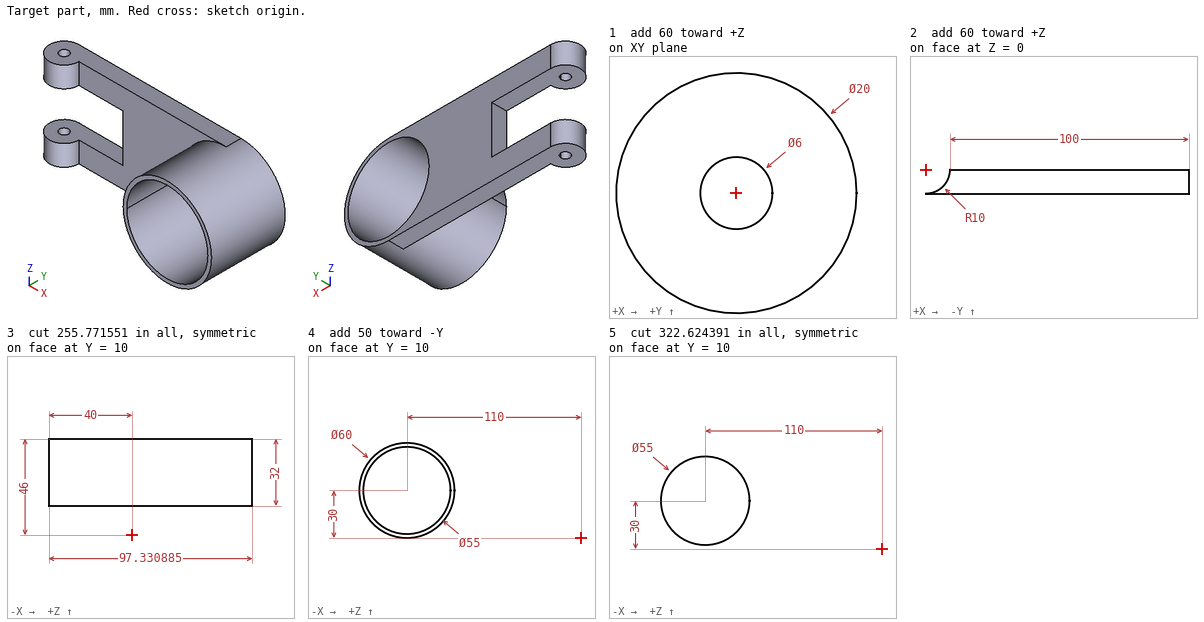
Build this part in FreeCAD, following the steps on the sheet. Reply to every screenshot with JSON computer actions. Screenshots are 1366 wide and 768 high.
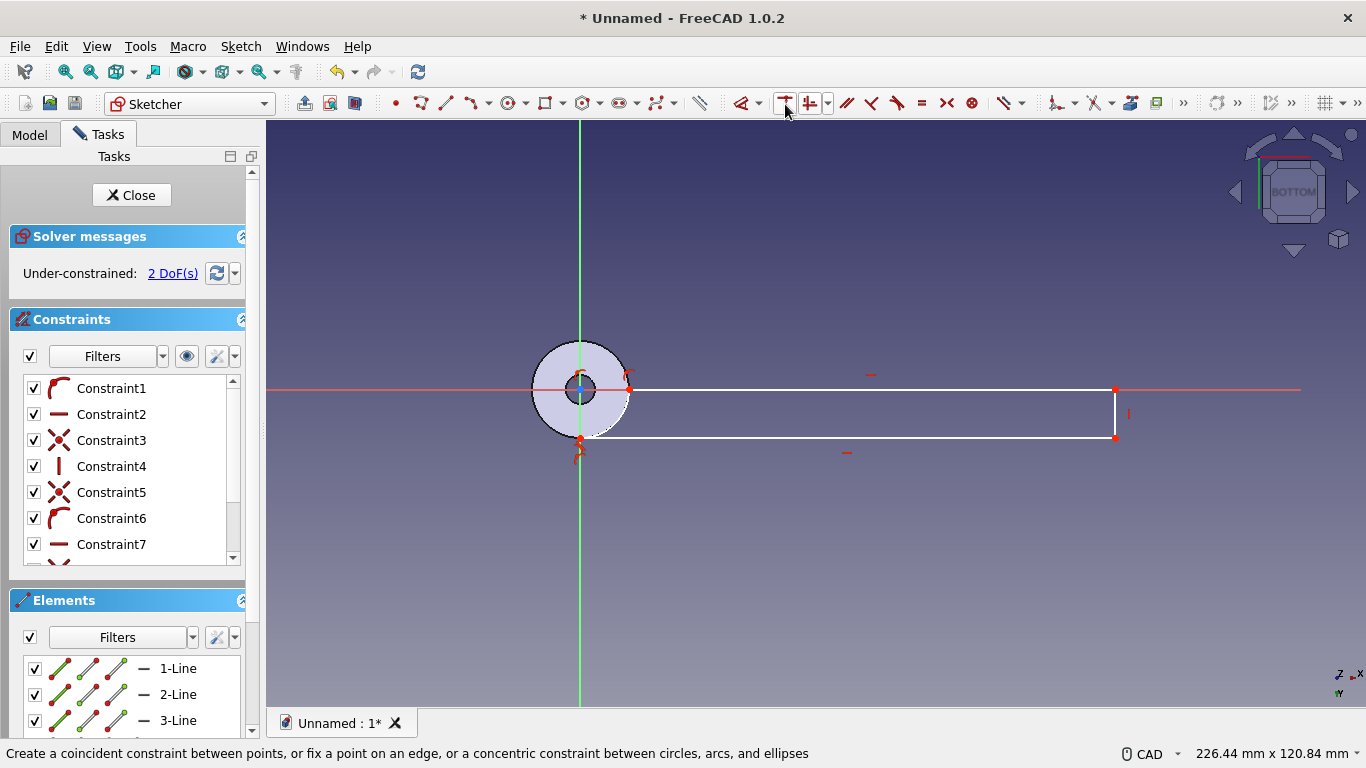
{"action": "left_click", "coordinate": [740, 104]}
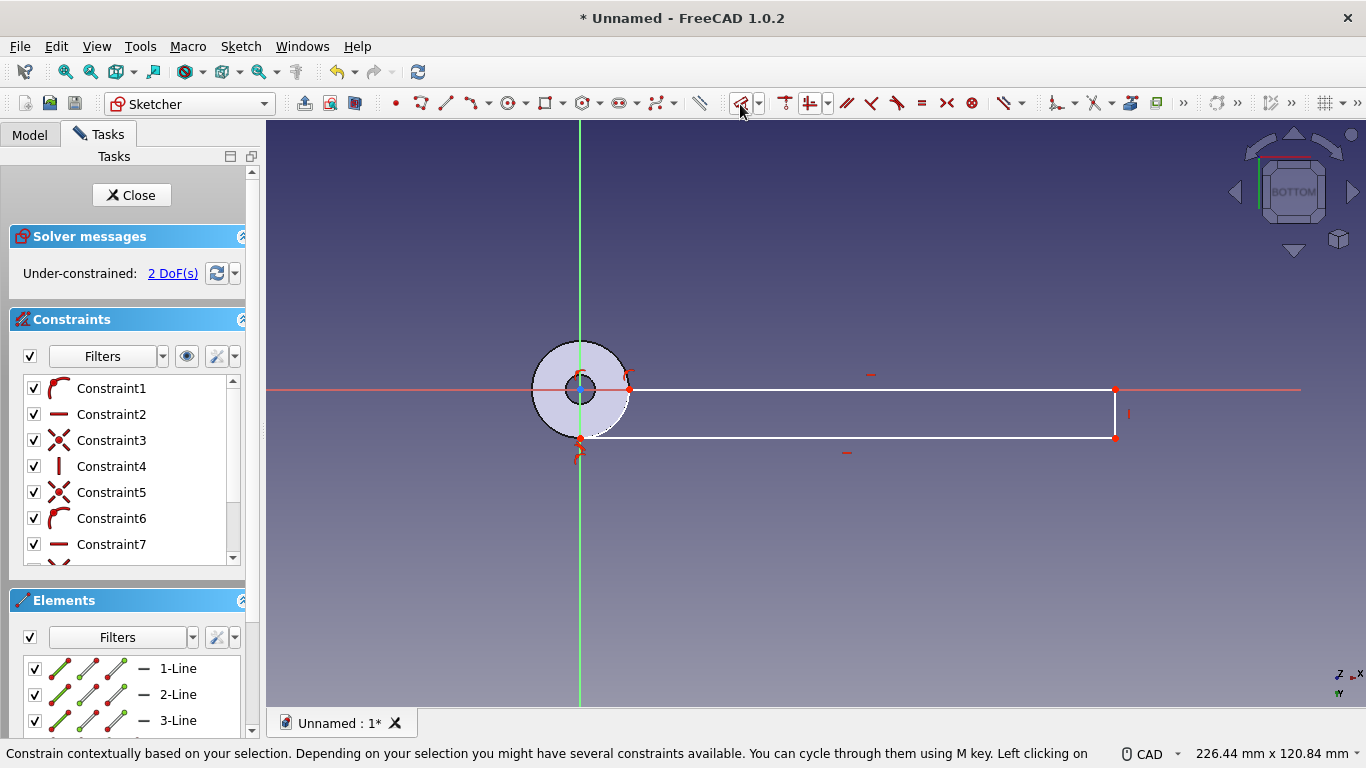
{"action": "left_click", "coordinate": [624, 412]}
{"action": "left_click", "coordinate": [626, 457]}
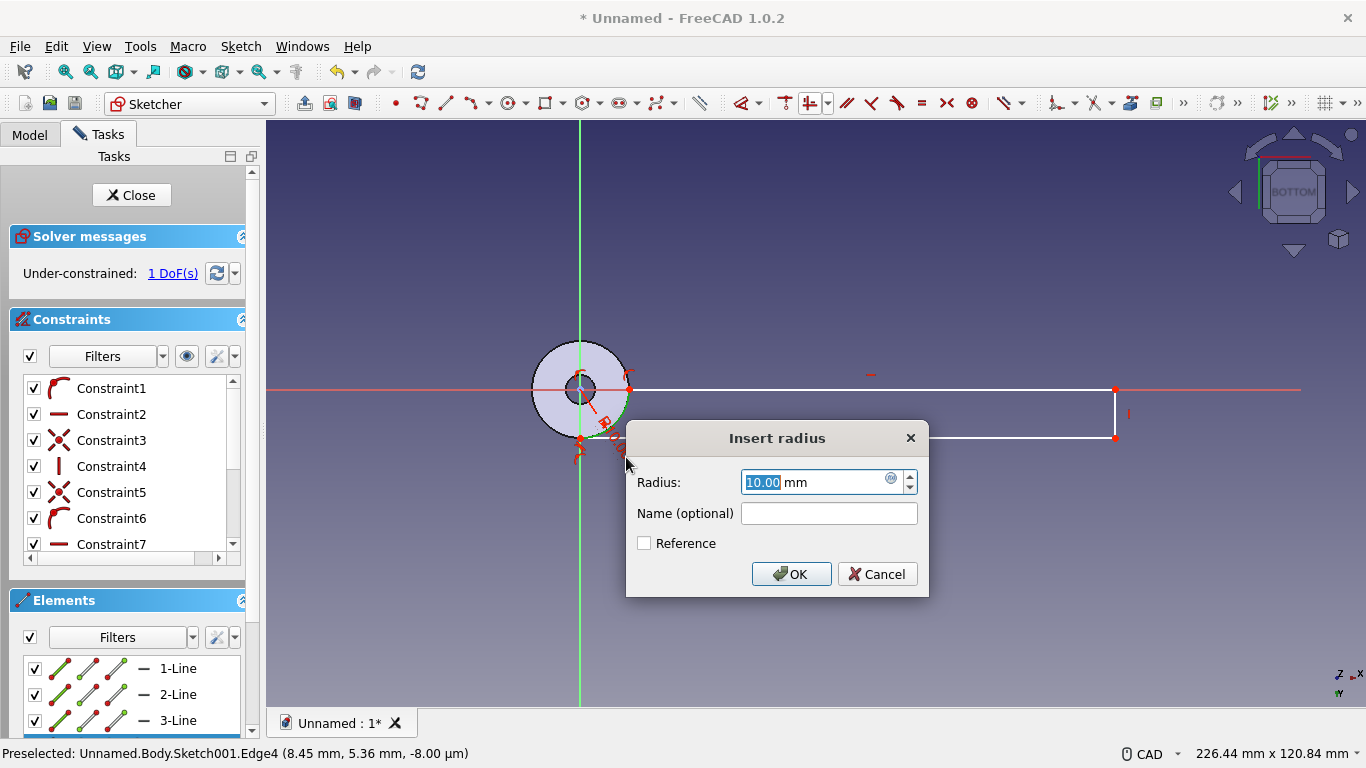
{"action": "type", "text": "10"}
{"action": "key", "text": "Return"}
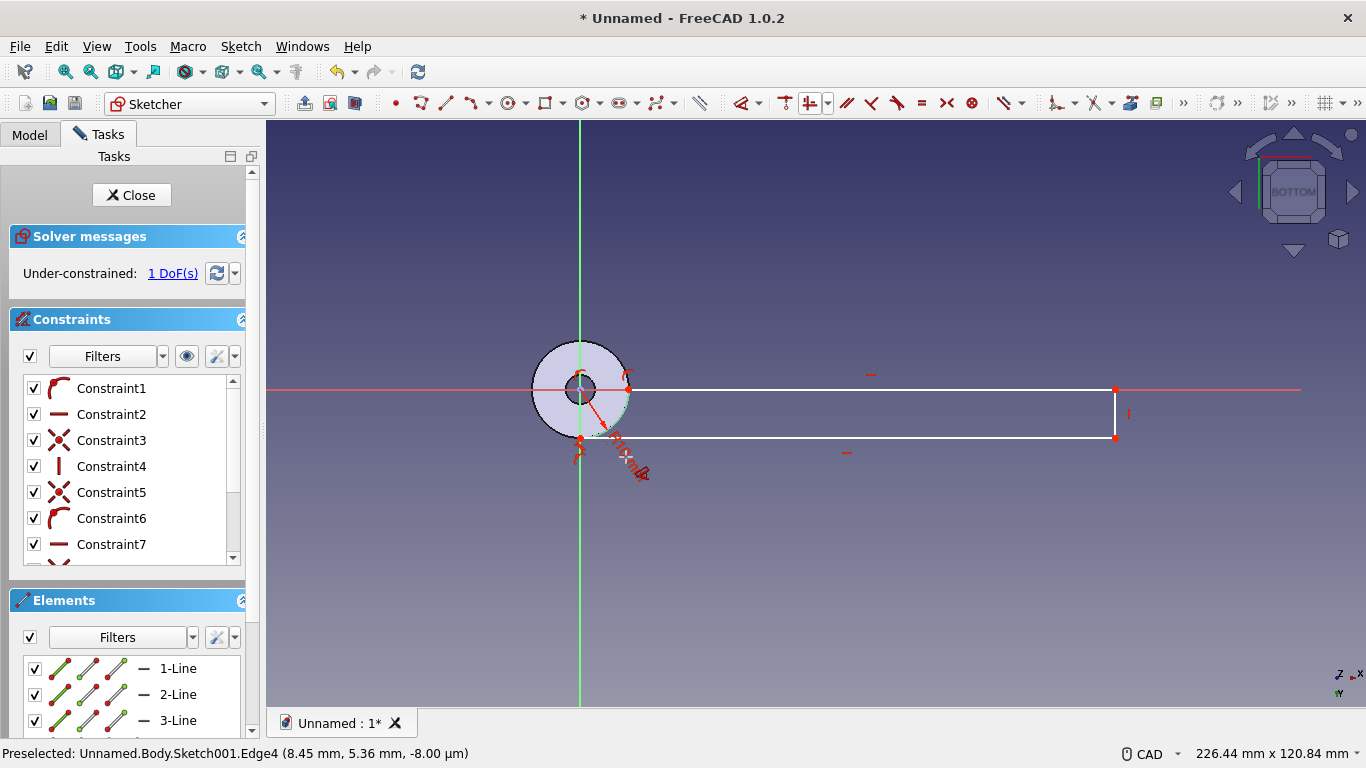
{"action": "left_click", "coordinate": [775, 390]}
{"action": "left_click", "coordinate": [872, 356]}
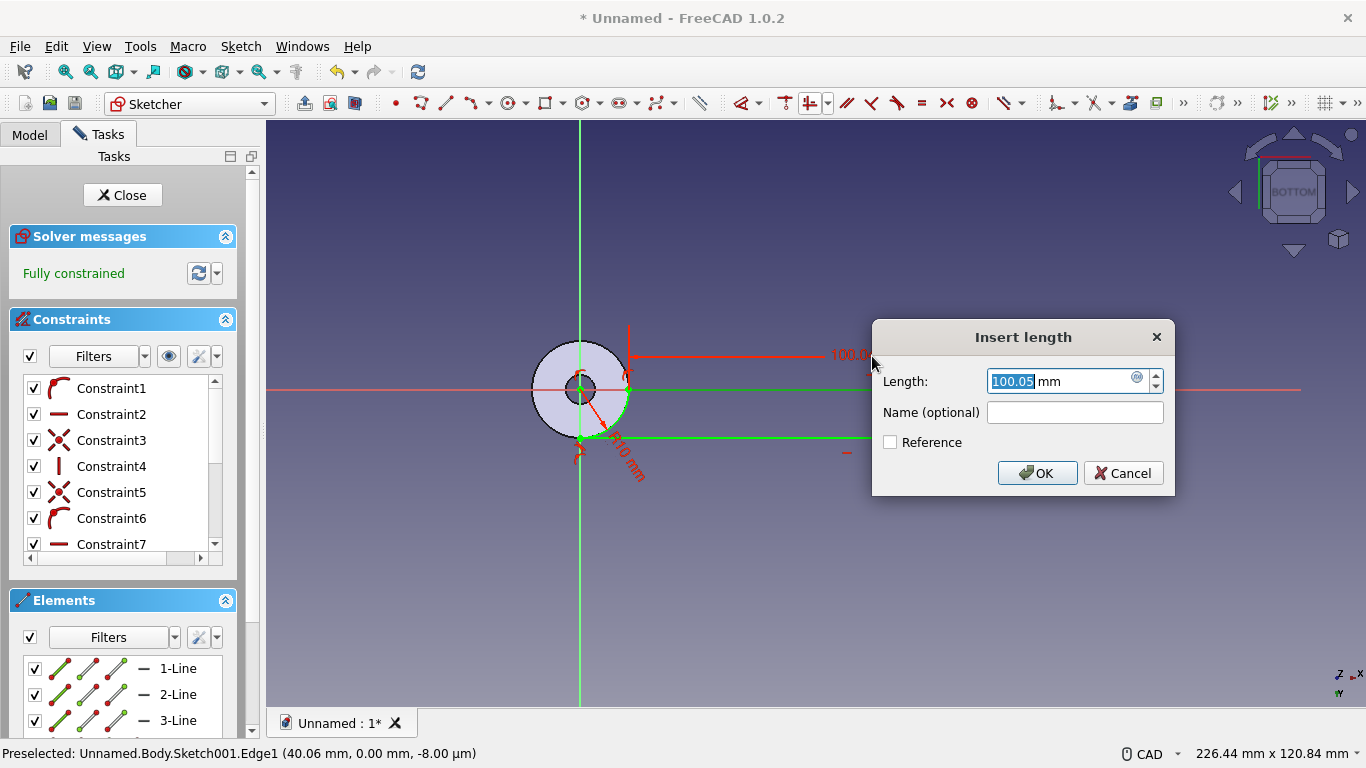
{"action": "type", "text": "100"}
{"action": "key", "text": "Return"}
{"action": "key", "text": "Escape"}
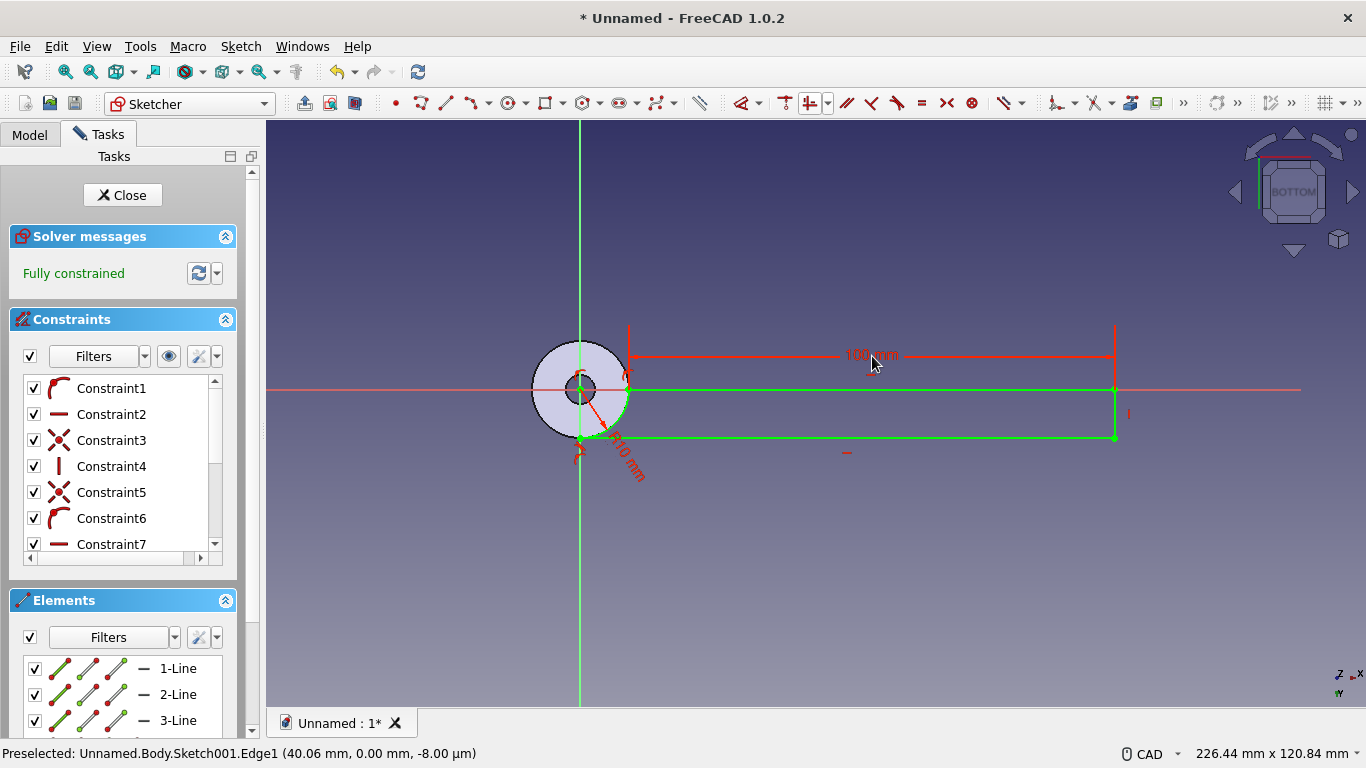
{"action": "left_click", "coordinate": [123, 195]}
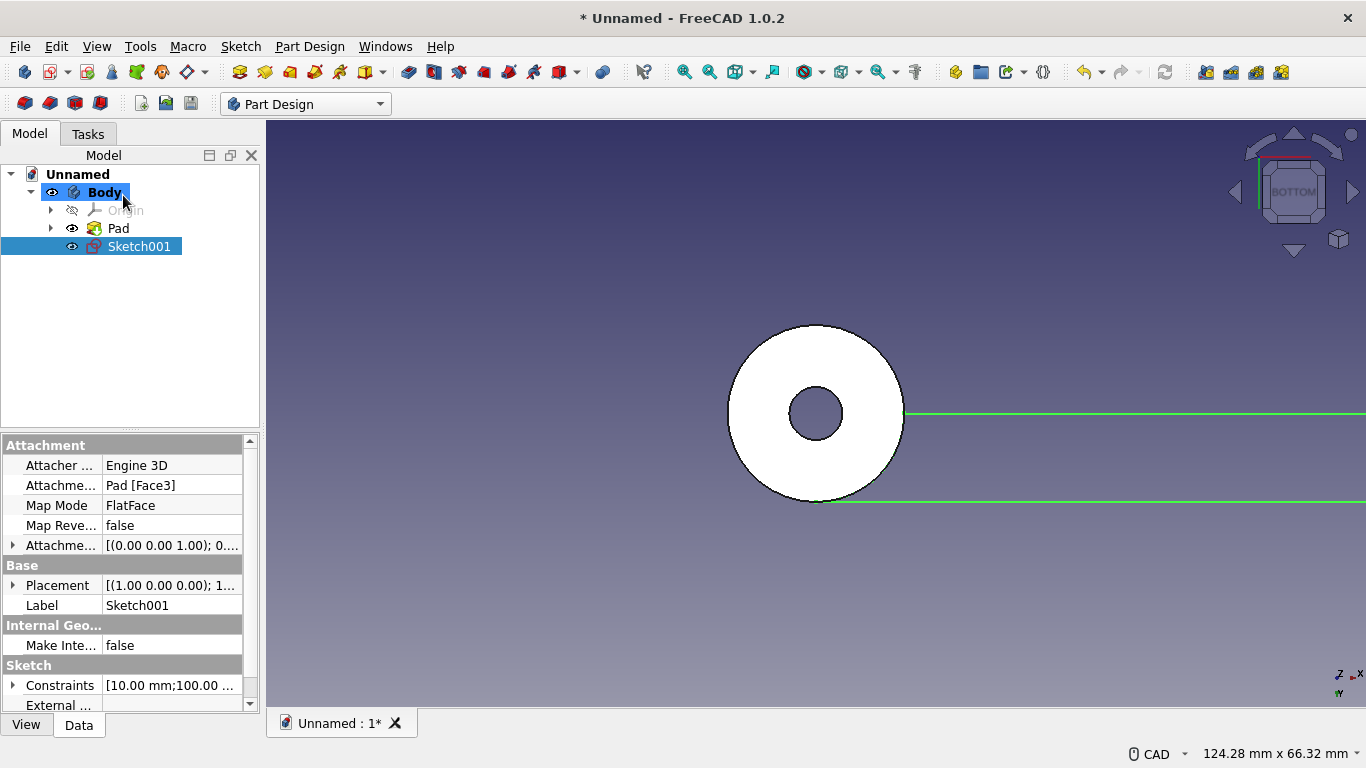
{"action": "left_click", "coordinate": [240, 72]}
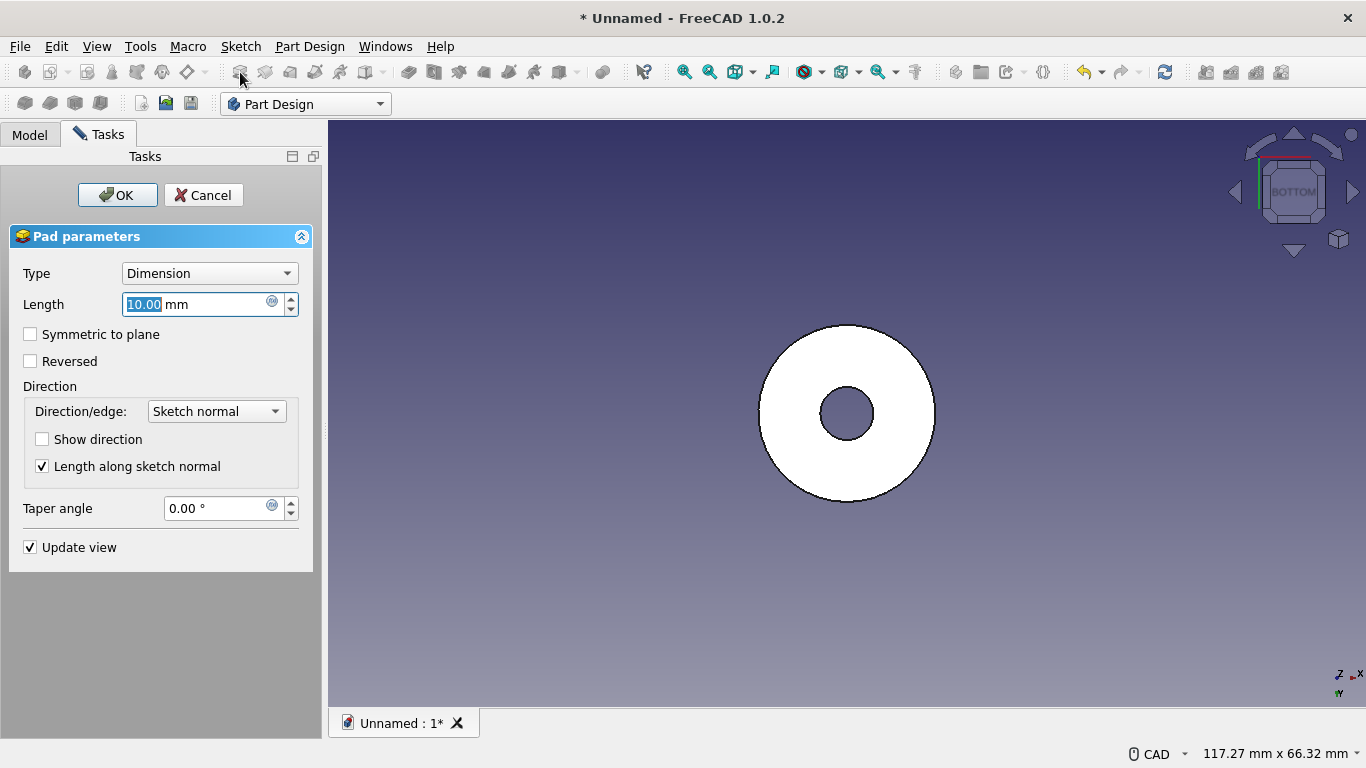
{"action": "type", "text": "60"}
{"action": "key", "text": "Tab"}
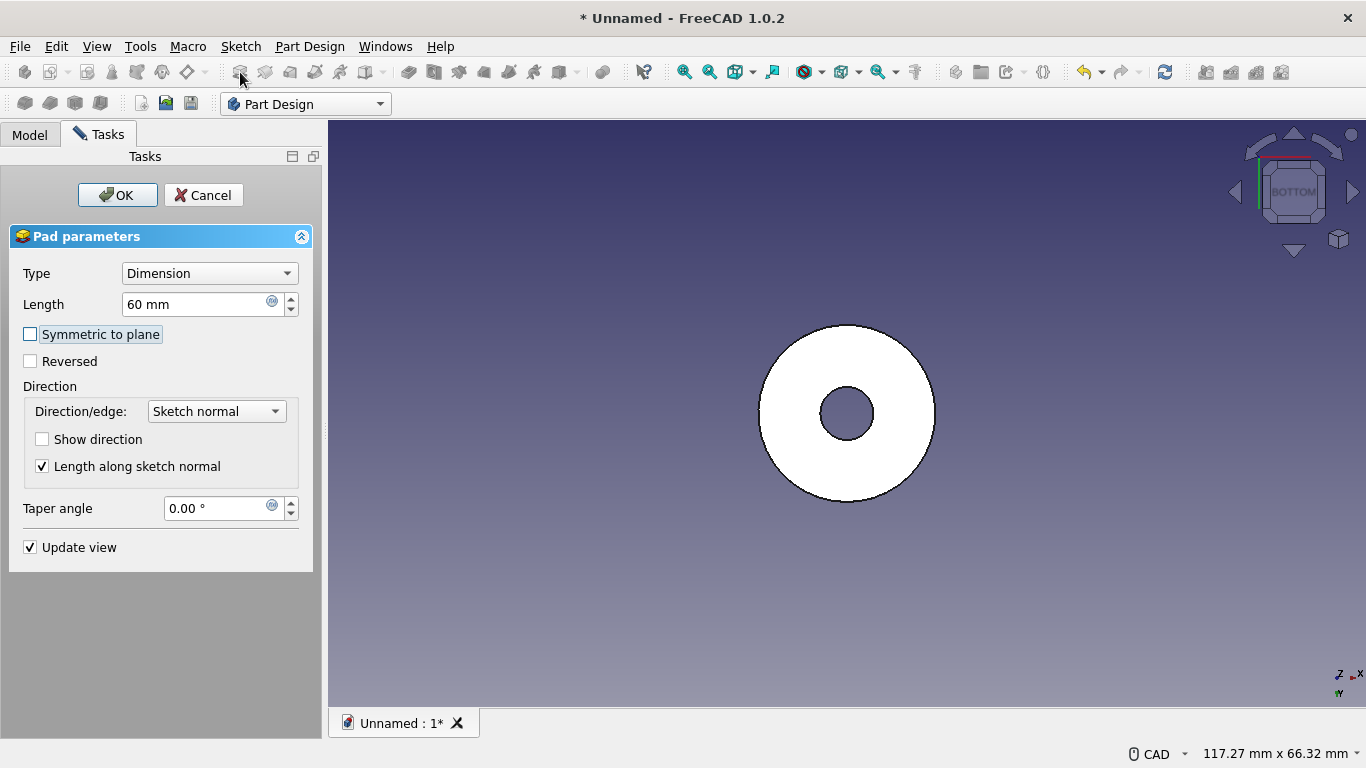
{"action": "left_click", "coordinate": [31, 361]}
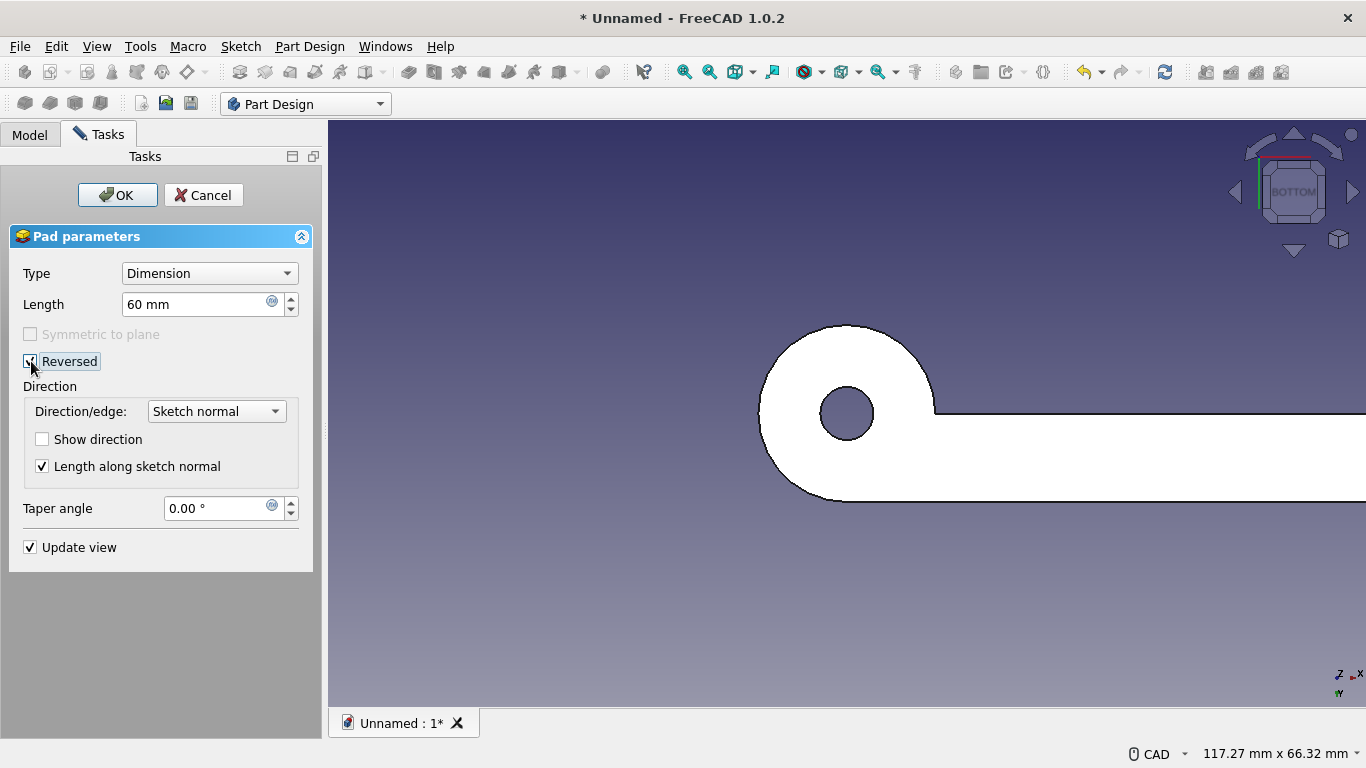
{"action": "left_click", "coordinate": [118, 195]}